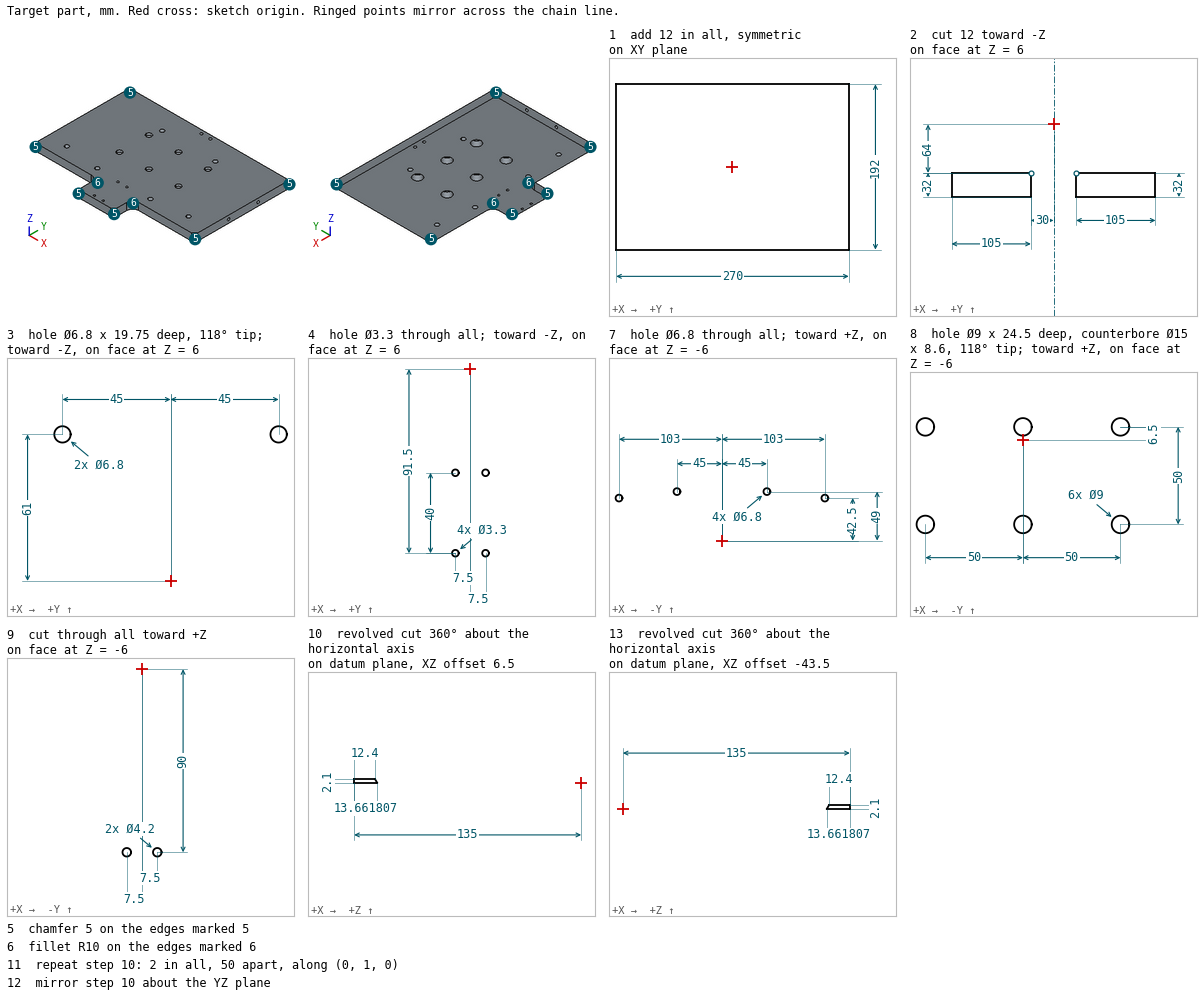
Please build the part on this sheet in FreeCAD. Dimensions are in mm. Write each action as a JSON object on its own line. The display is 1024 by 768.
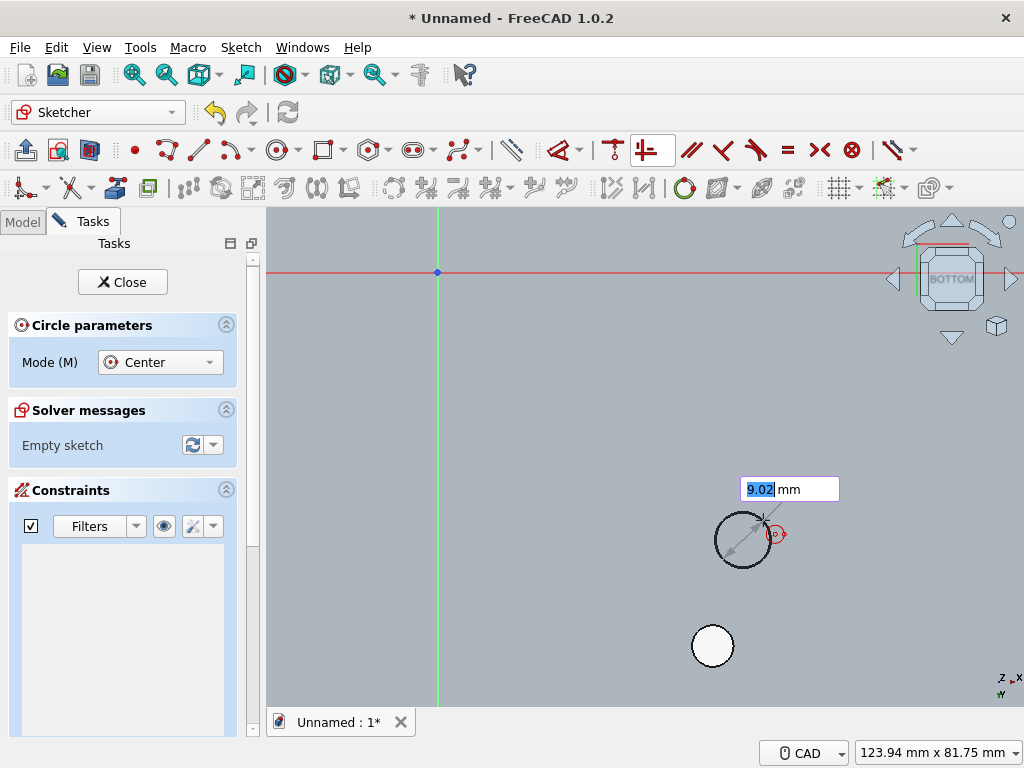
{"action": "type", "text": "9"}
{"action": "key", "text": "Return"}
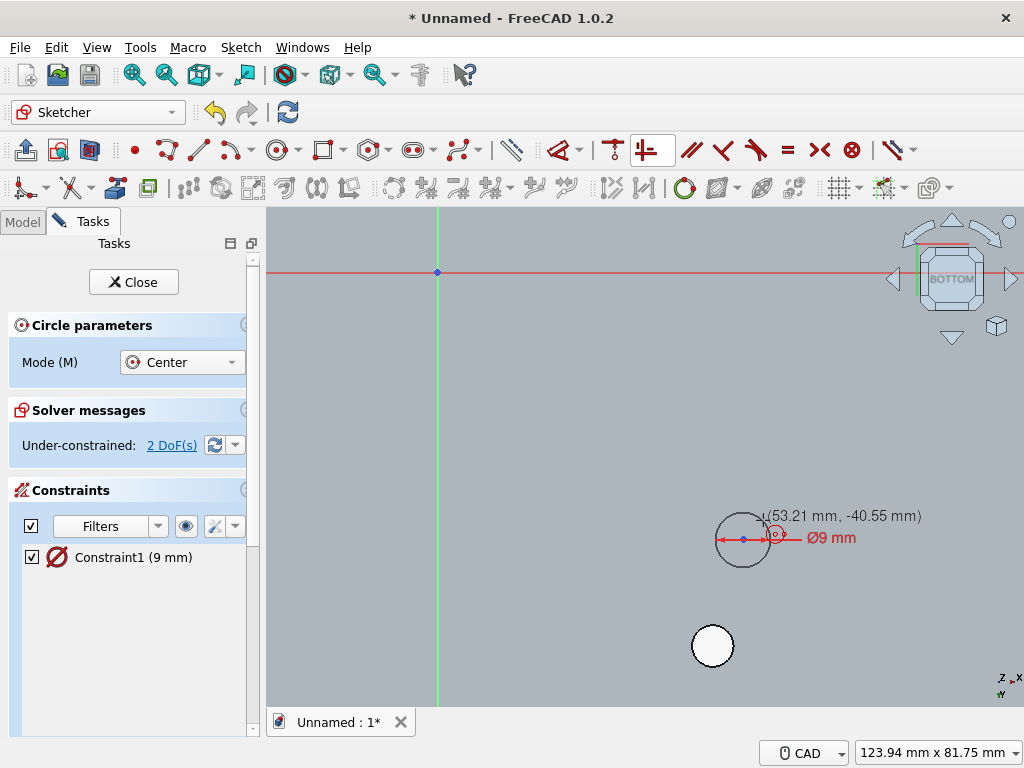
{"action": "scroll", "coordinate": [745, 543], "scroll_direction": "down", "scroll_amount": 3}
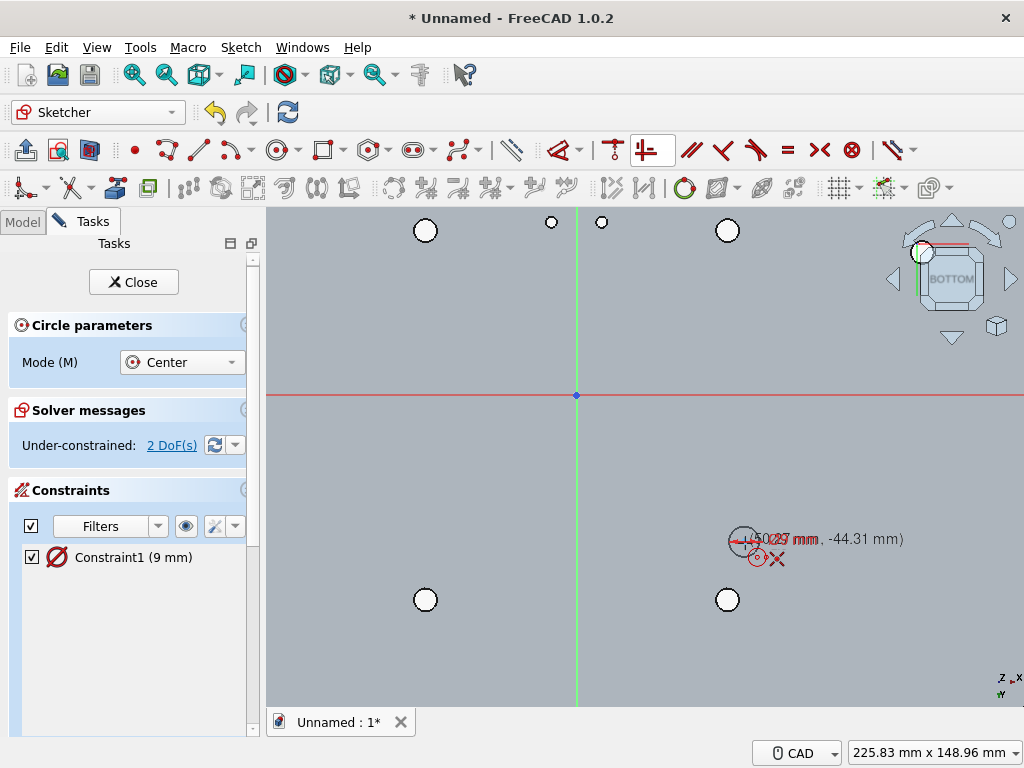
{"action": "scroll", "coordinate": [744, 373], "scroll_direction": "up", "scroll_amount": 3}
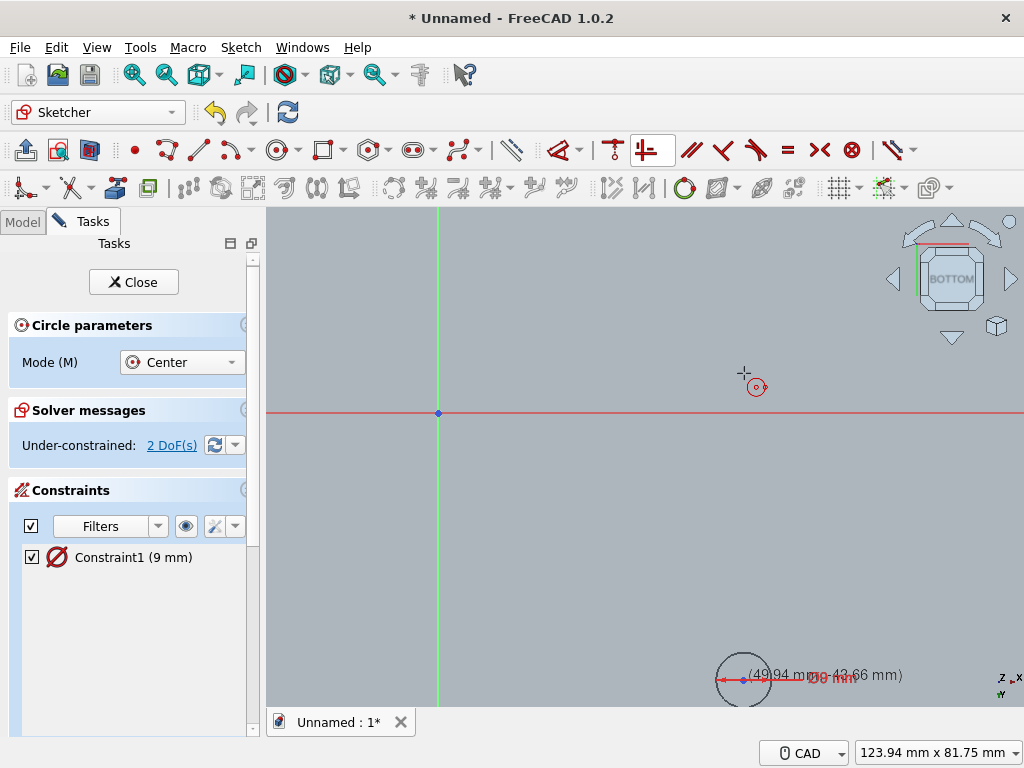
{"action": "left_click", "coordinate": [744, 373]}
{"action": "mouse_move", "coordinate": [764, 354]}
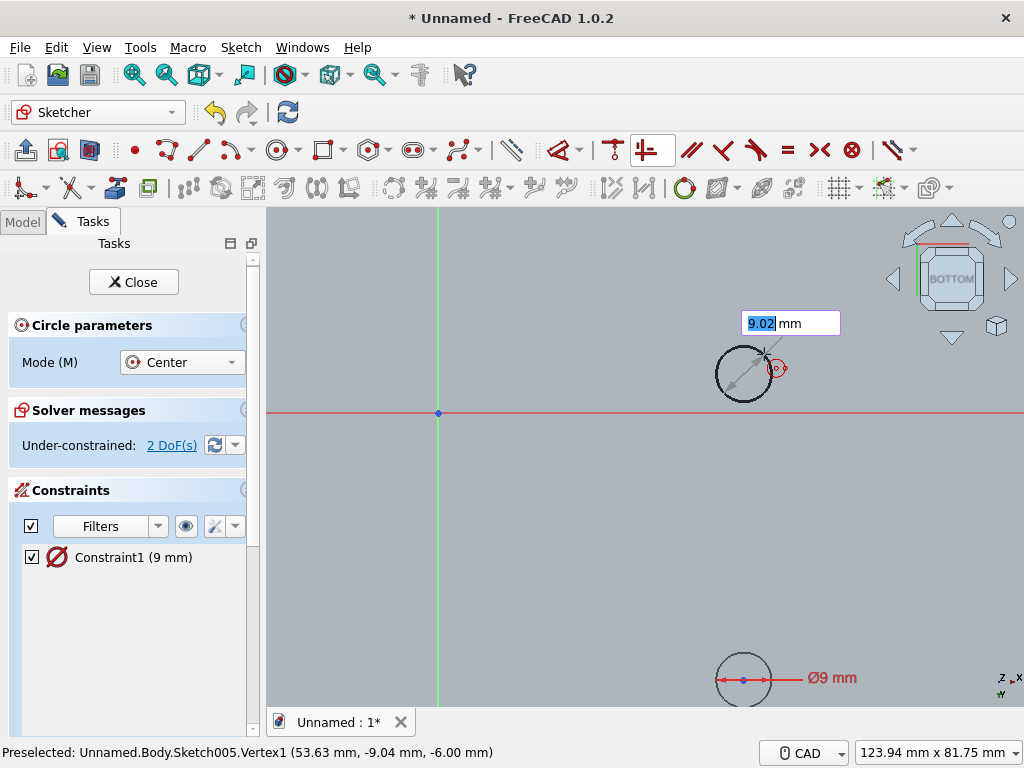
{"action": "type", "text": "9"}
{"action": "key", "text": "Return"}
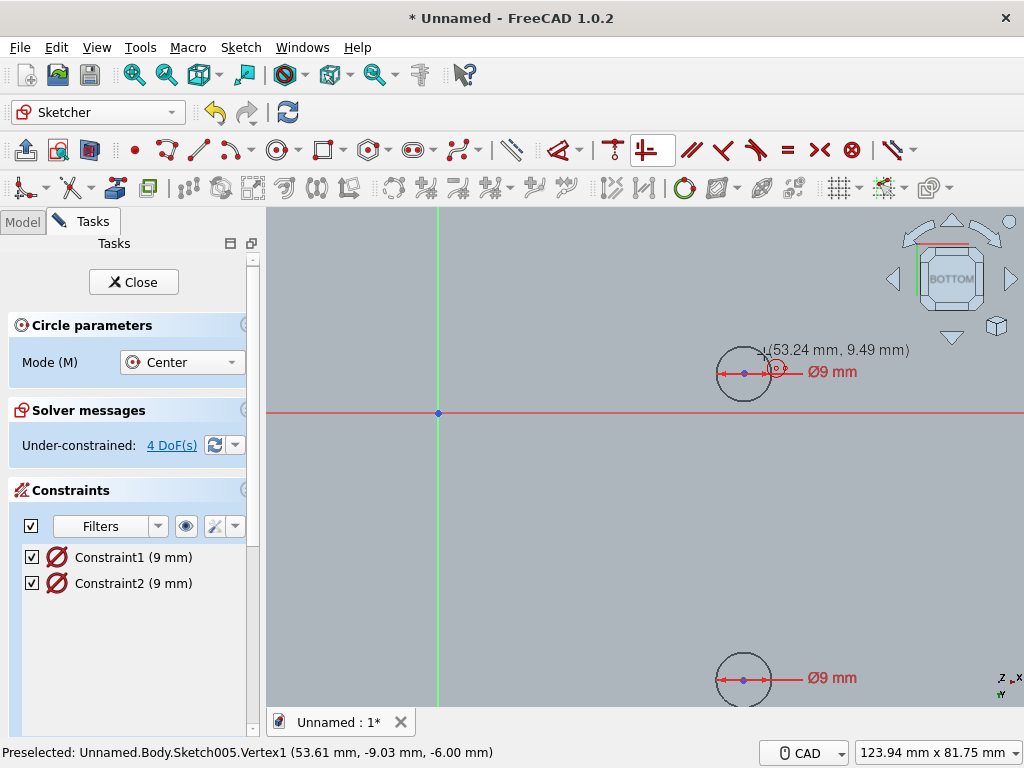
{"action": "scroll", "coordinate": [744, 373], "scroll_direction": "down", "scroll_amount": 3}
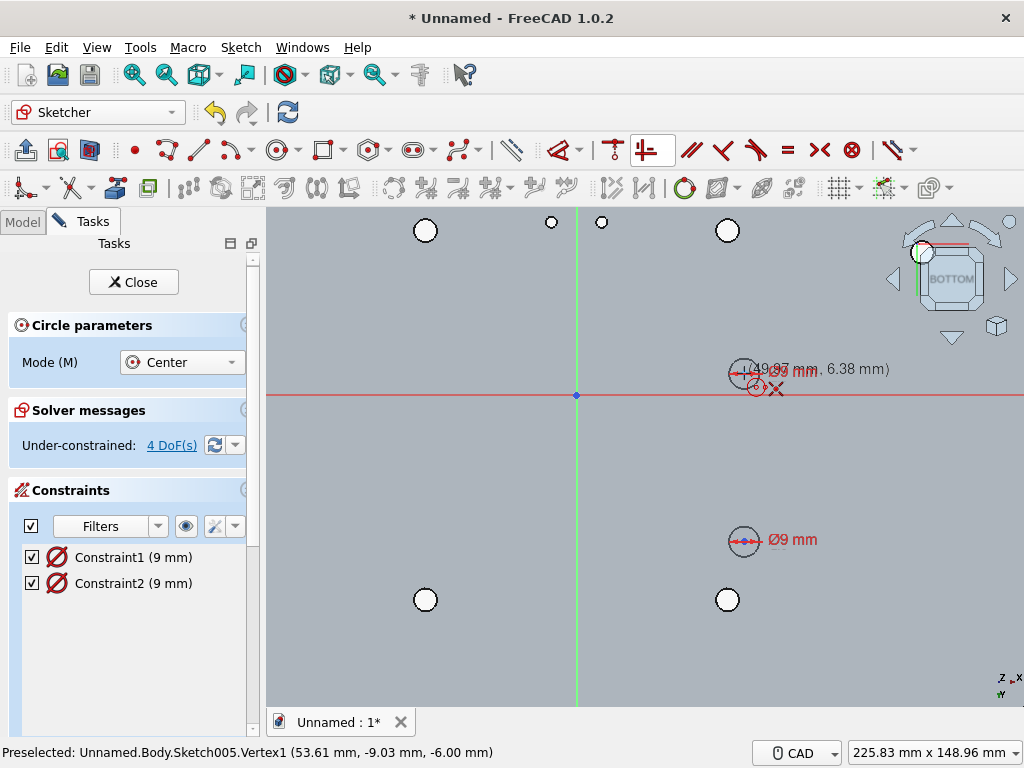
{"action": "scroll", "coordinate": [577, 541], "scroll_direction": "up", "scroll_amount": 3}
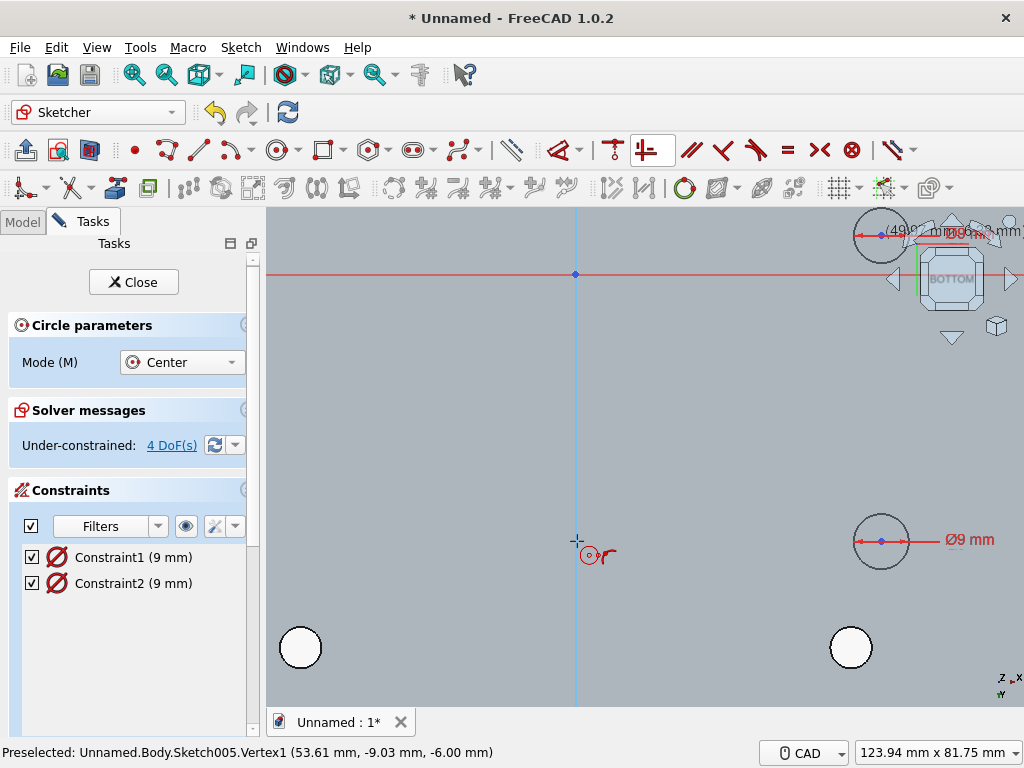
{"action": "left_click", "coordinate": [576, 541]}
{"action": "mouse_move", "coordinate": [595, 521]}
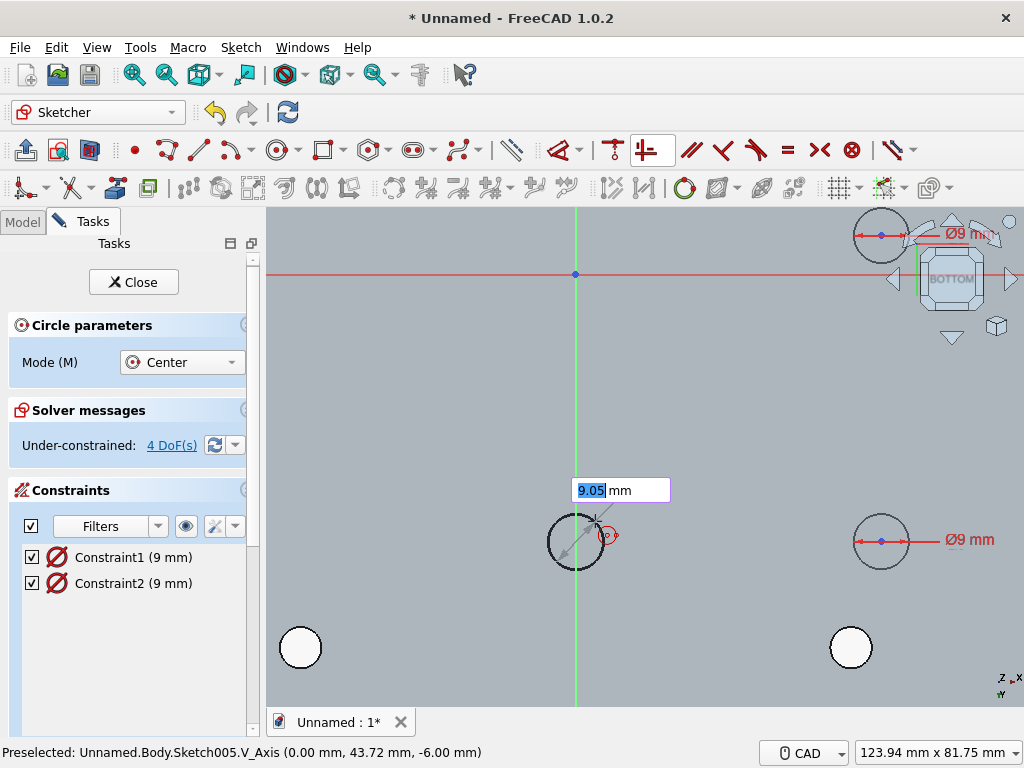
{"action": "type", "text": "9"}
{"action": "key", "text": "Return"}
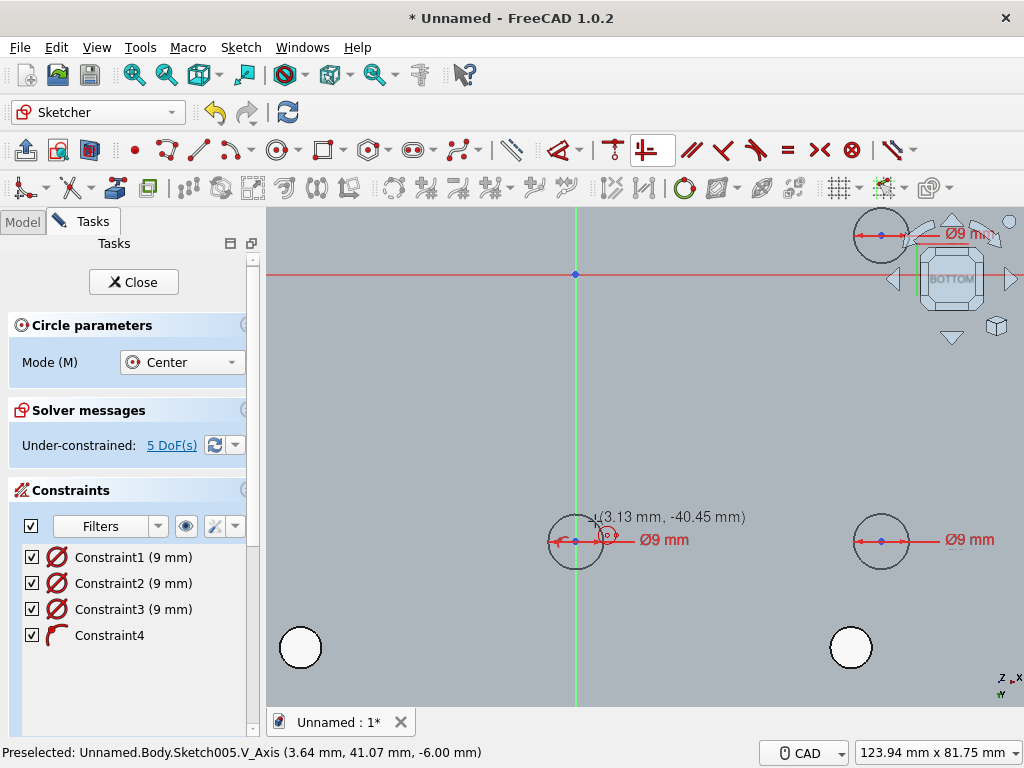
{"action": "scroll", "coordinate": [577, 541], "scroll_direction": "down", "scroll_amount": 3}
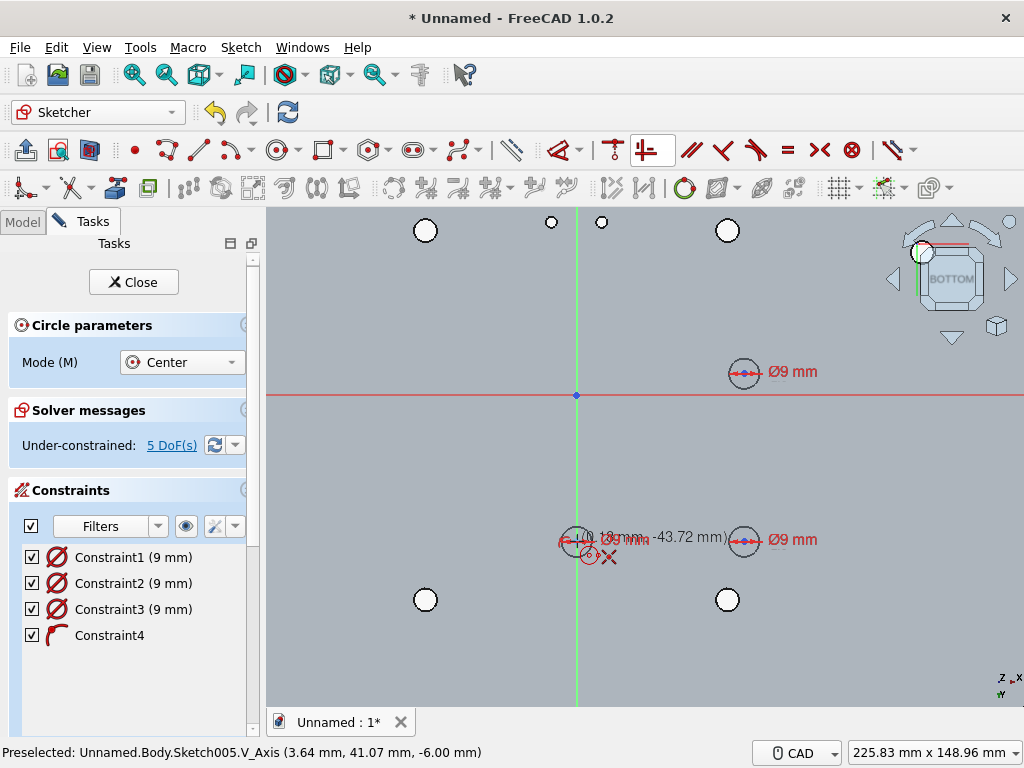
{"action": "scroll", "coordinate": [577, 373], "scroll_direction": "up", "scroll_amount": 3}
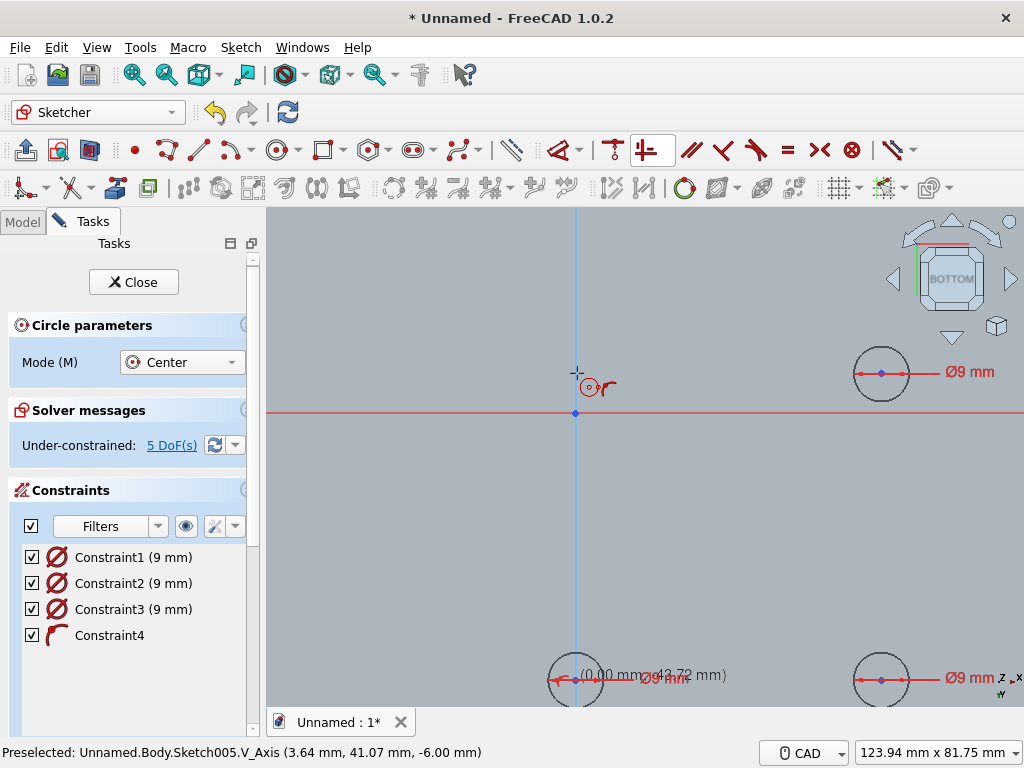
{"action": "left_click", "coordinate": [576, 373]}
{"action": "mouse_move", "coordinate": [595, 354]}